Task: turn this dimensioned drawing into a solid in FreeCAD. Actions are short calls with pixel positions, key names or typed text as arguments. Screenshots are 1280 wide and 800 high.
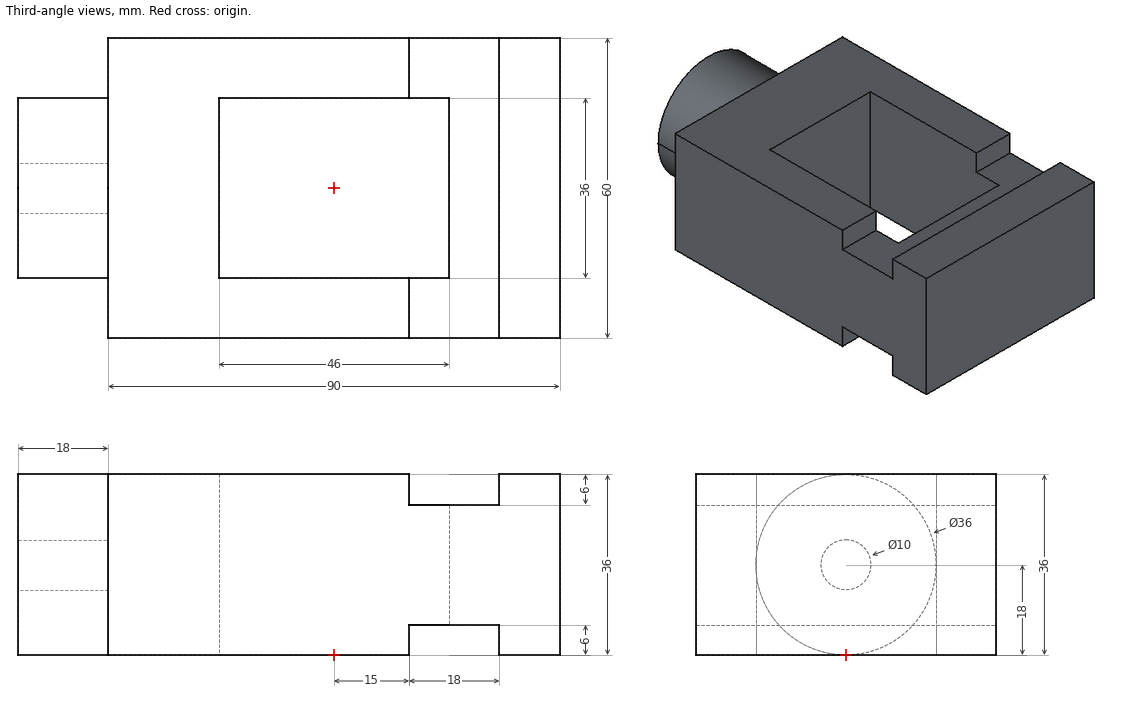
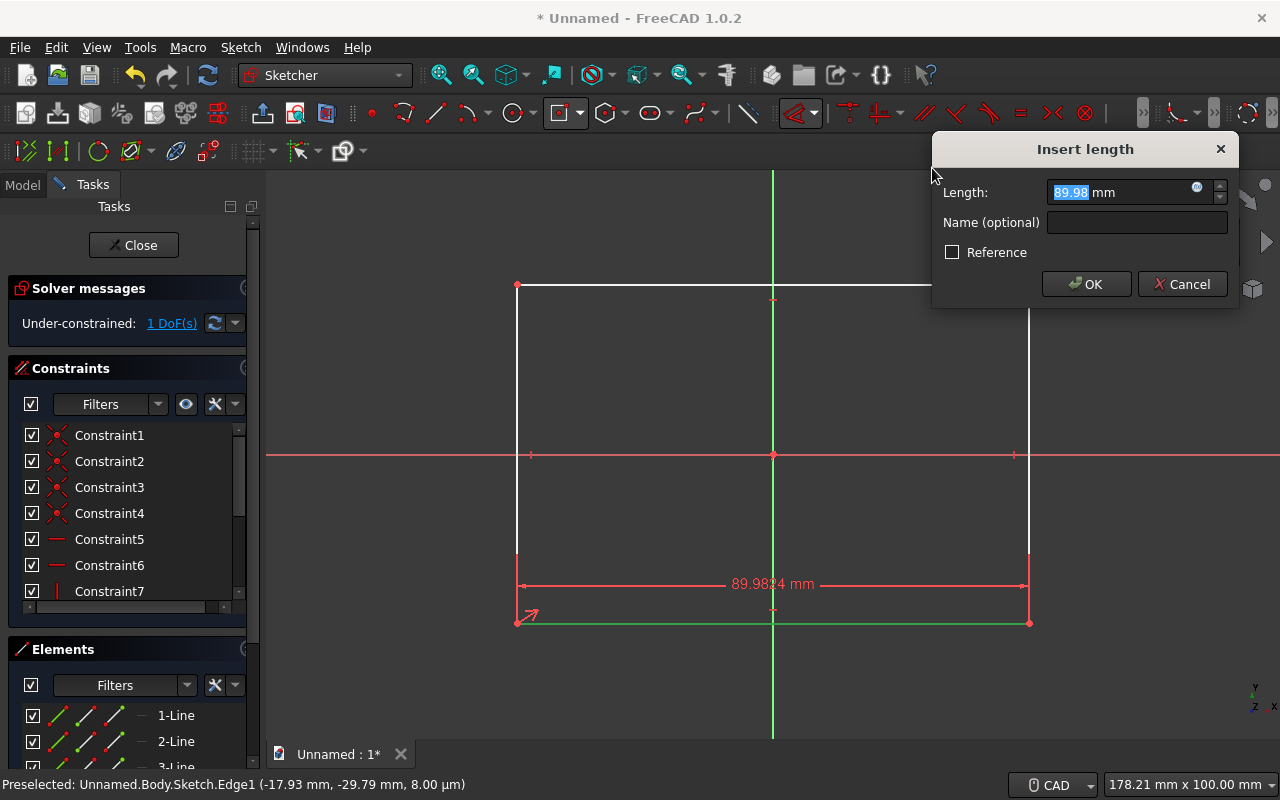
text(90)
key(Return)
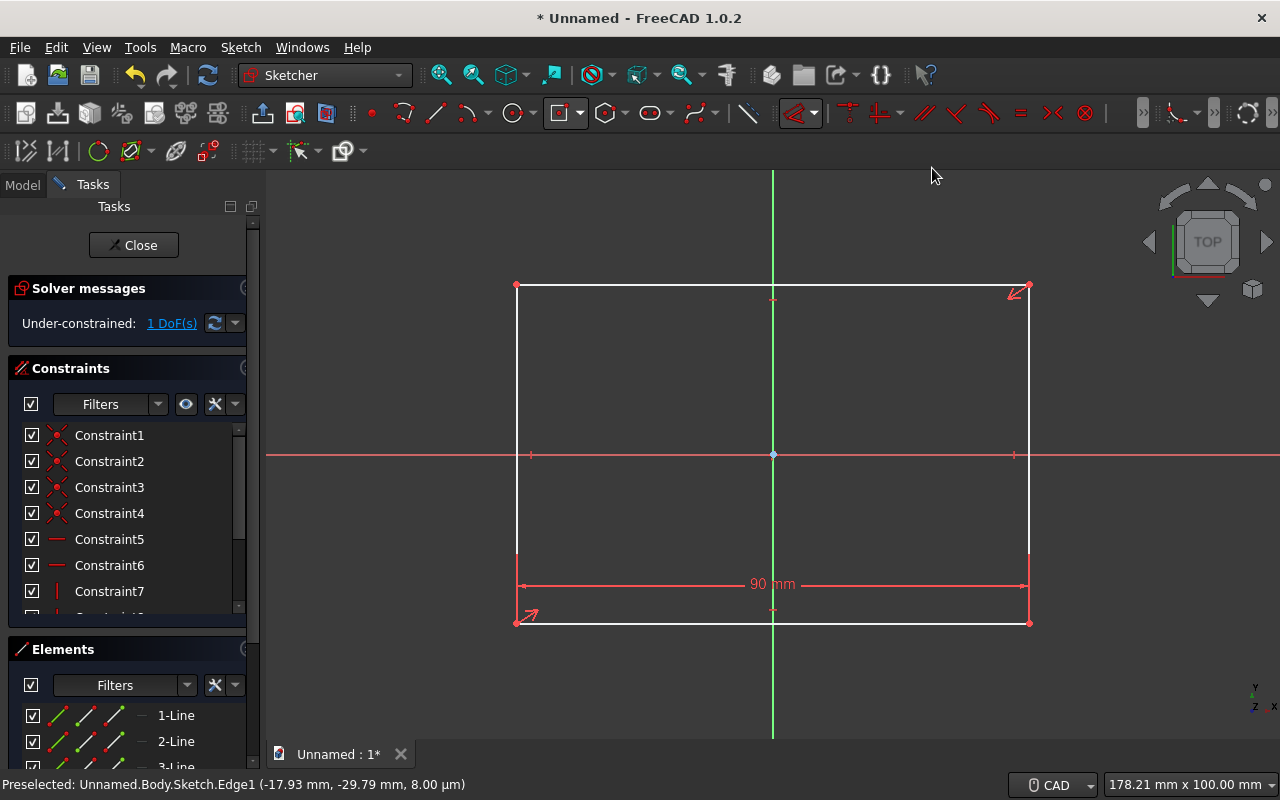
click(1029, 522)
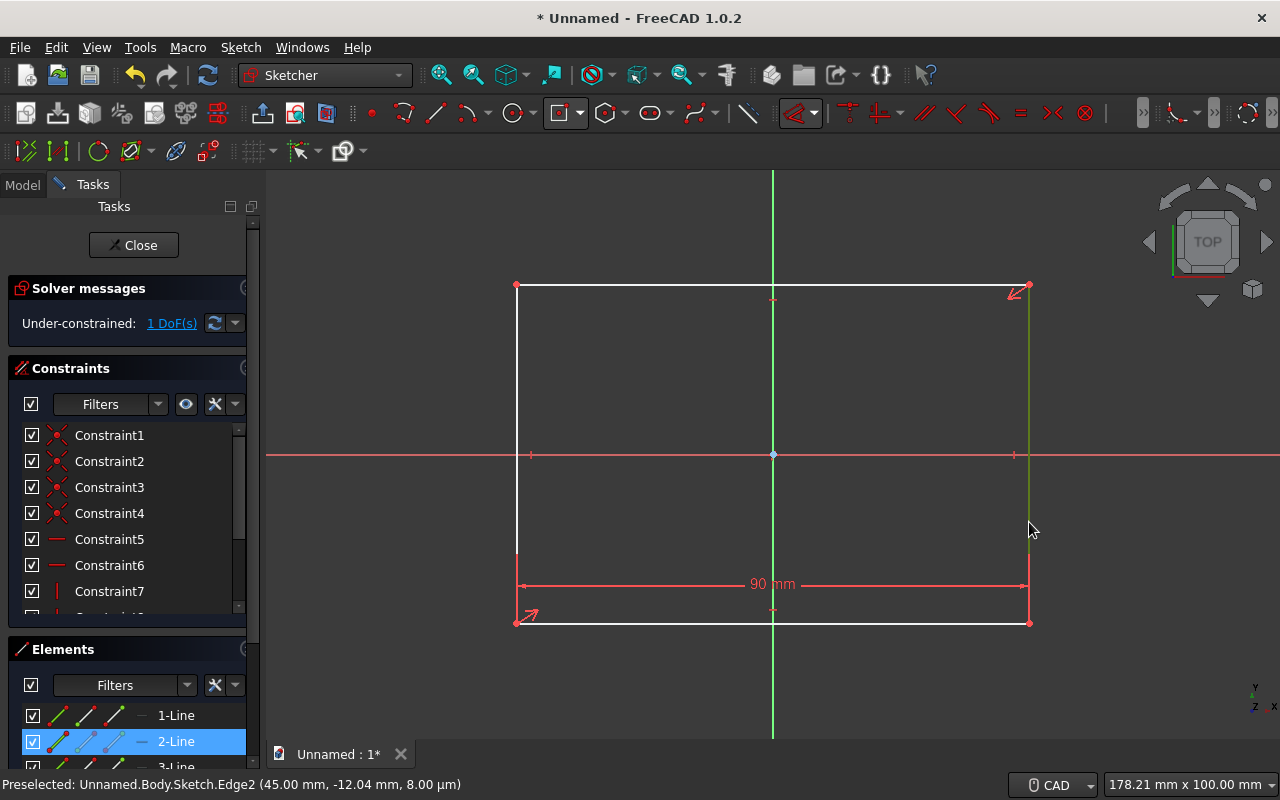
click(816, 114)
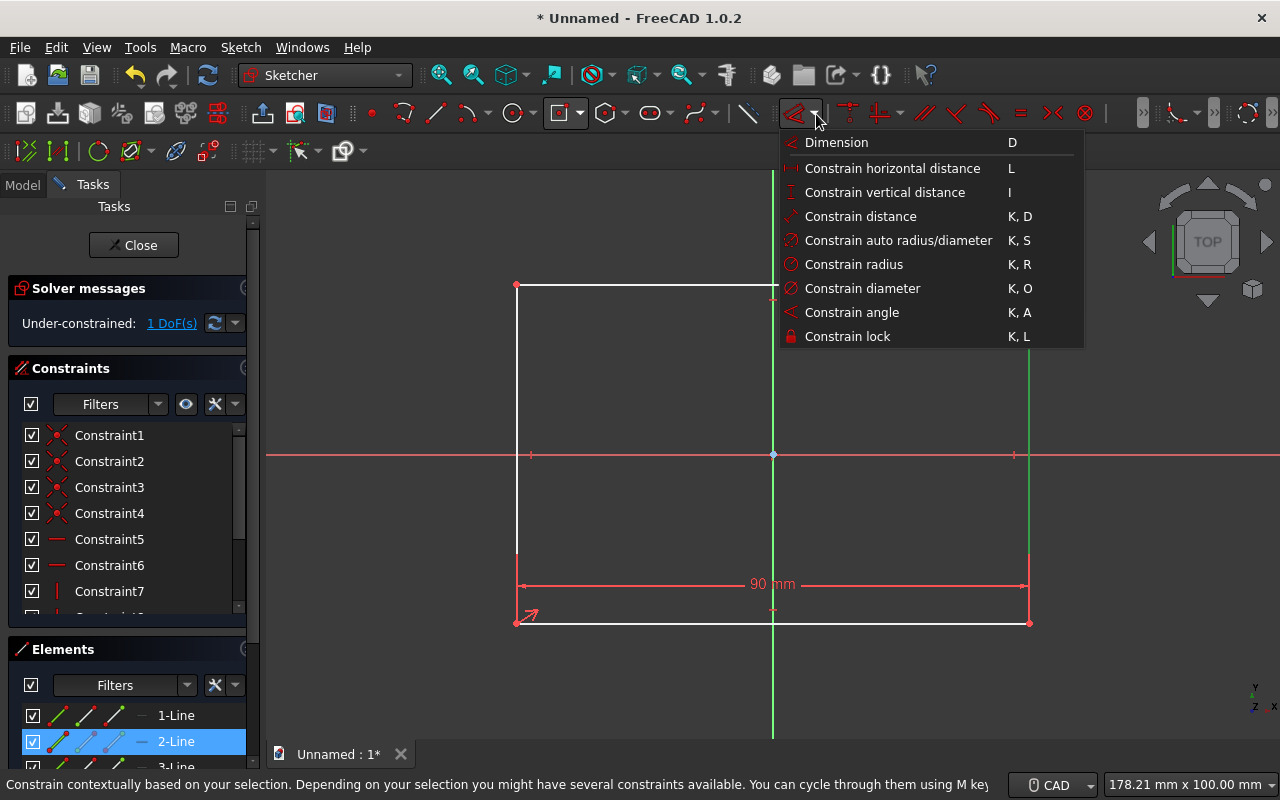
click(932, 192)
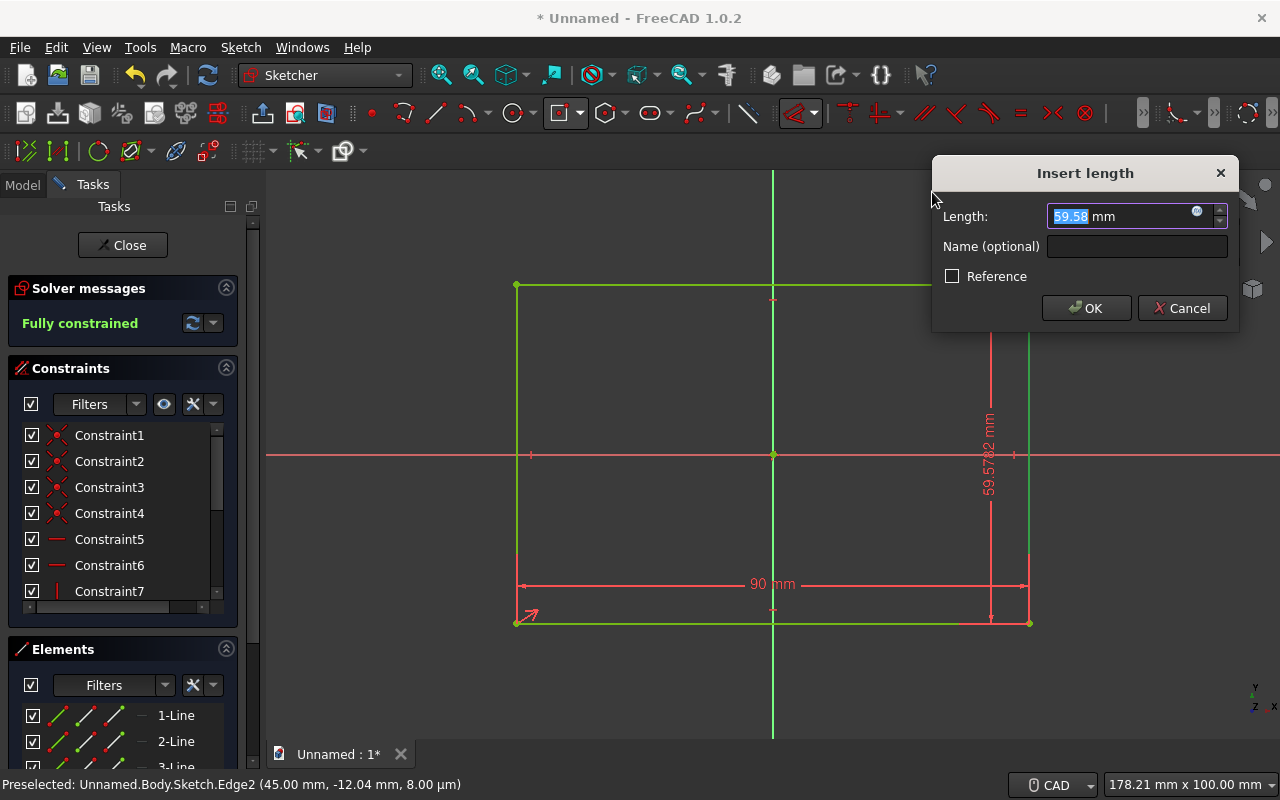
text(60)
key(Return)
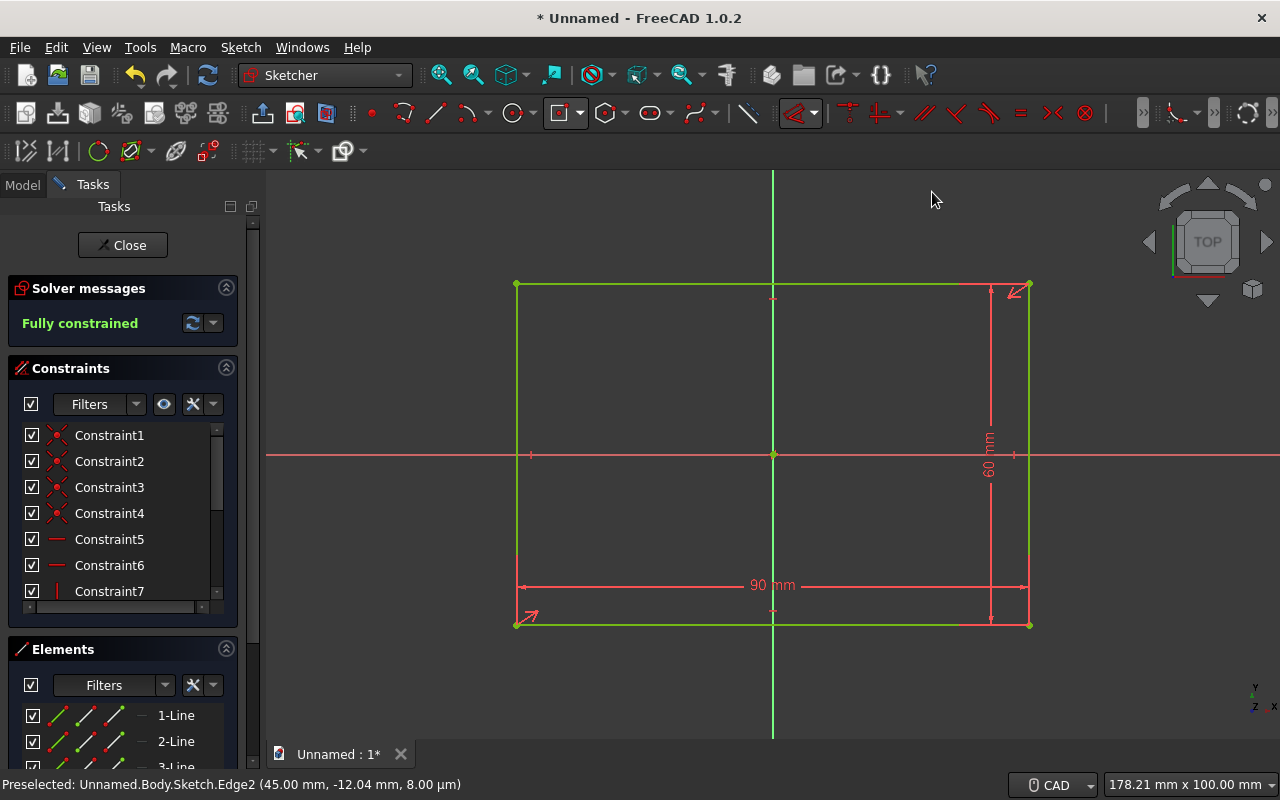
click(123, 245)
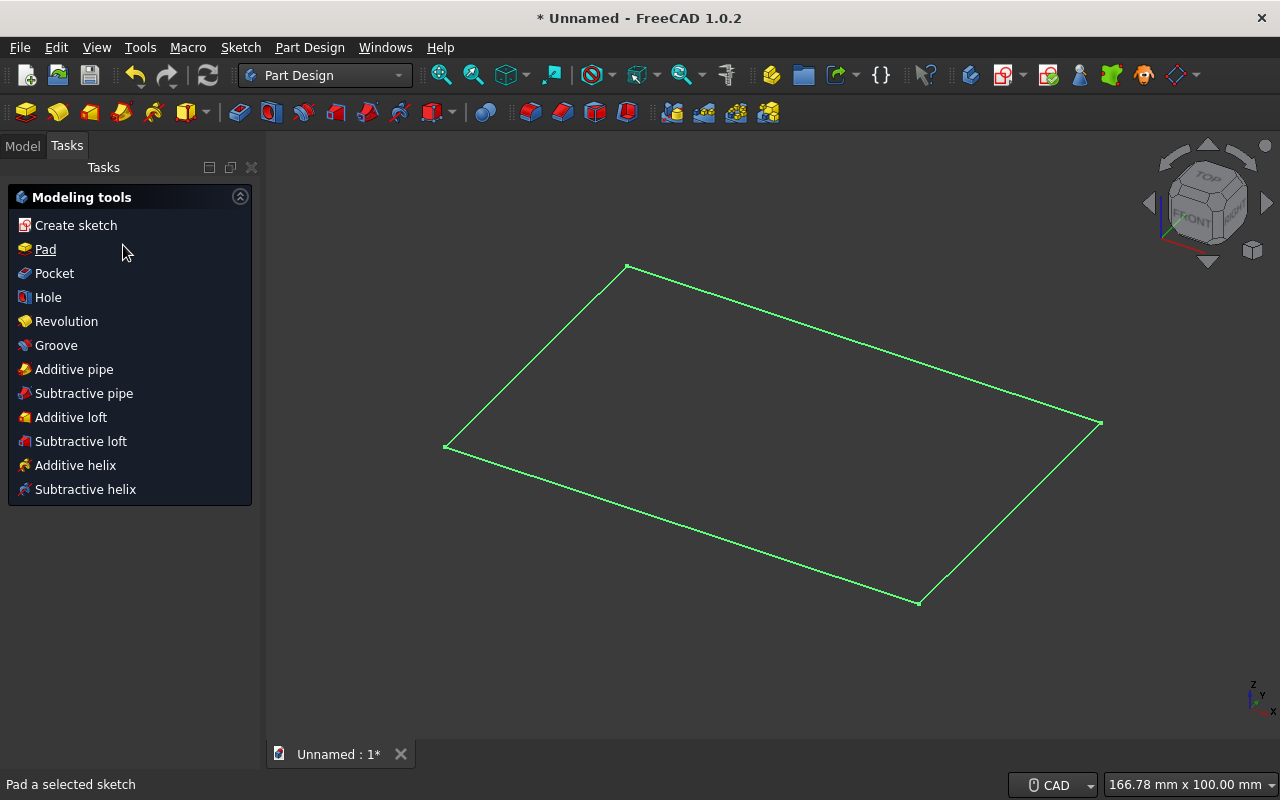
click(26, 112)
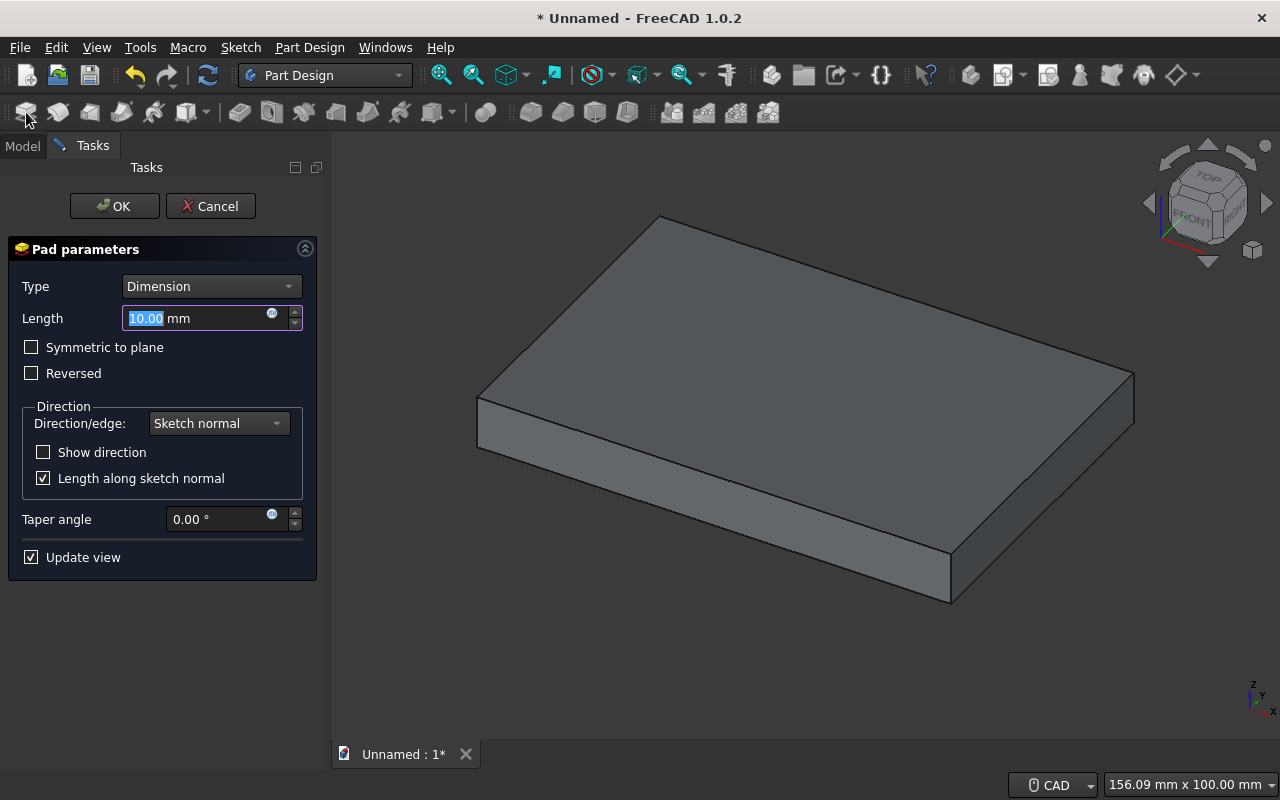
text(36)
key(Tab)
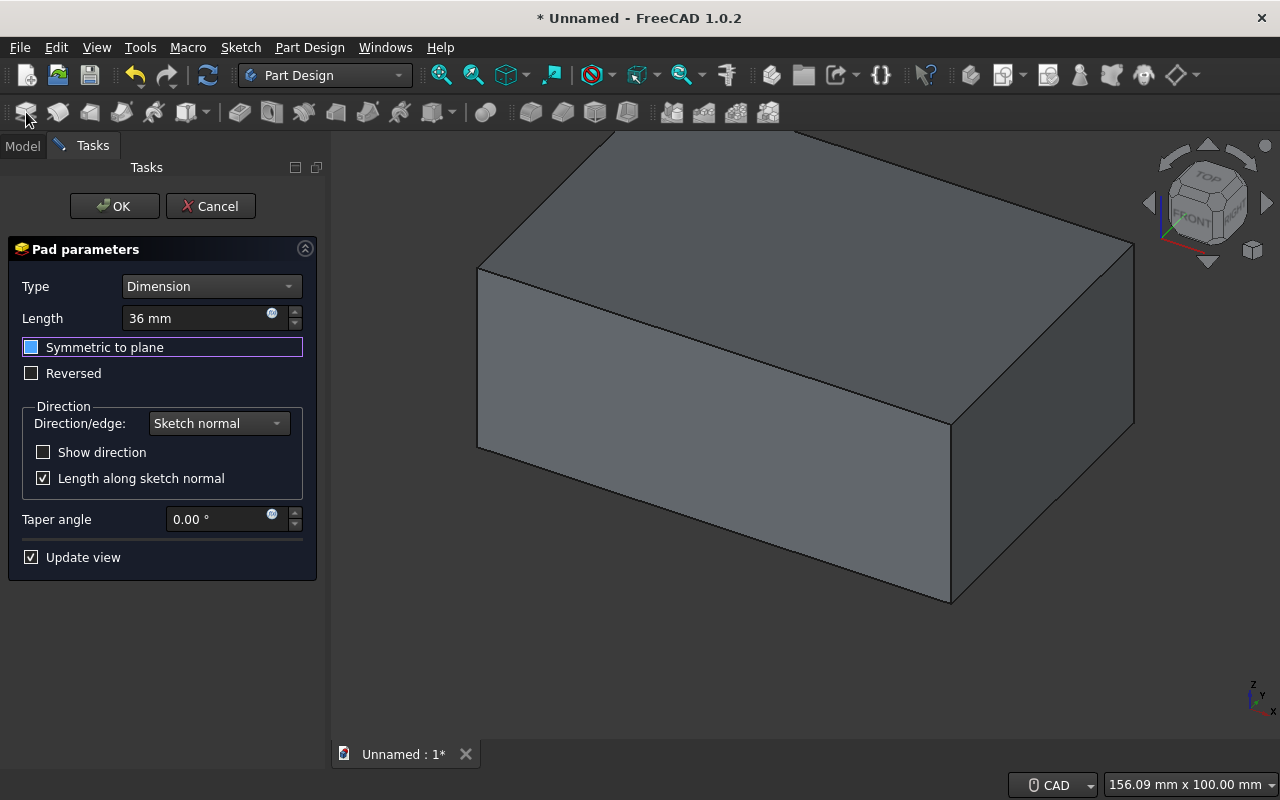
click(115, 206)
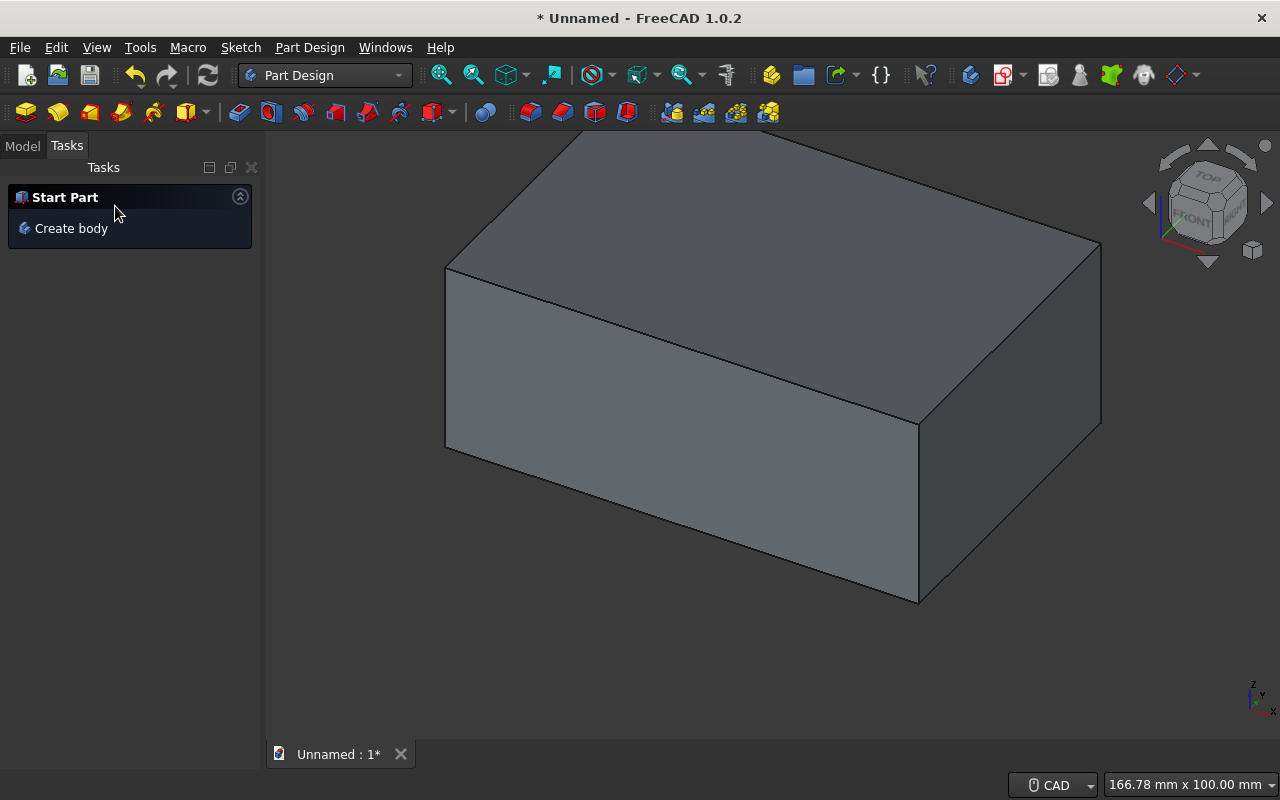
click(442, 76)